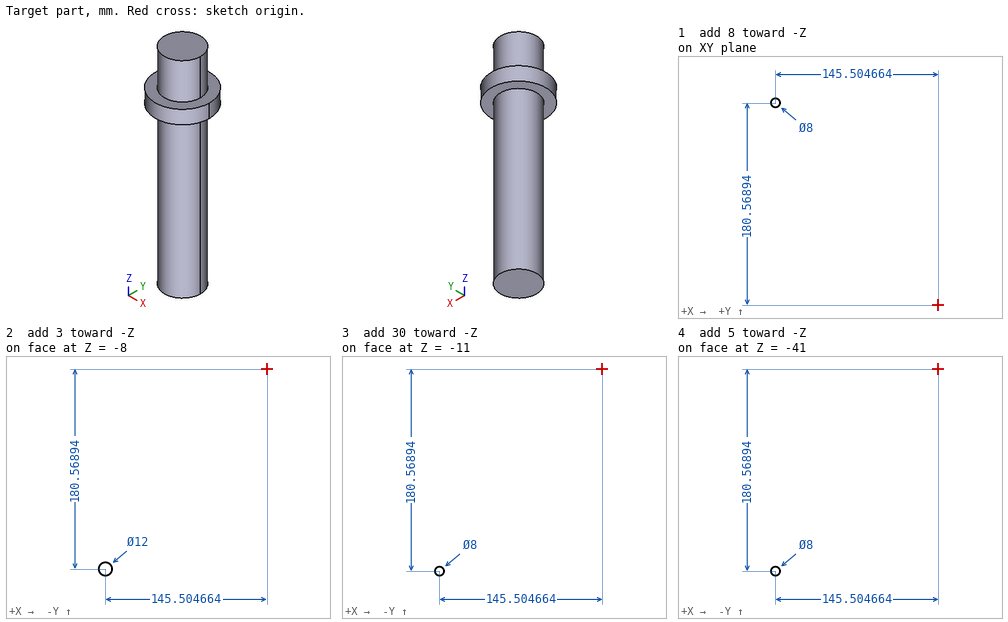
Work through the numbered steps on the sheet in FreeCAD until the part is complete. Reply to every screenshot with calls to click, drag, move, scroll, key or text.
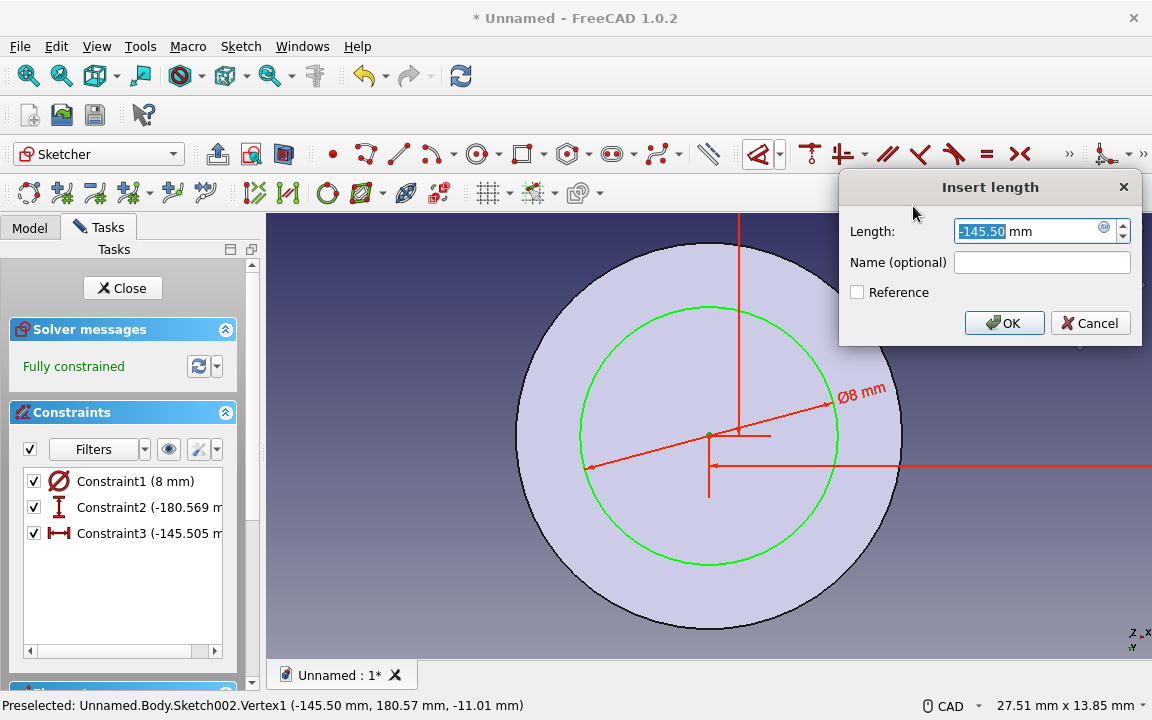
text(-145.504664)
key(Return)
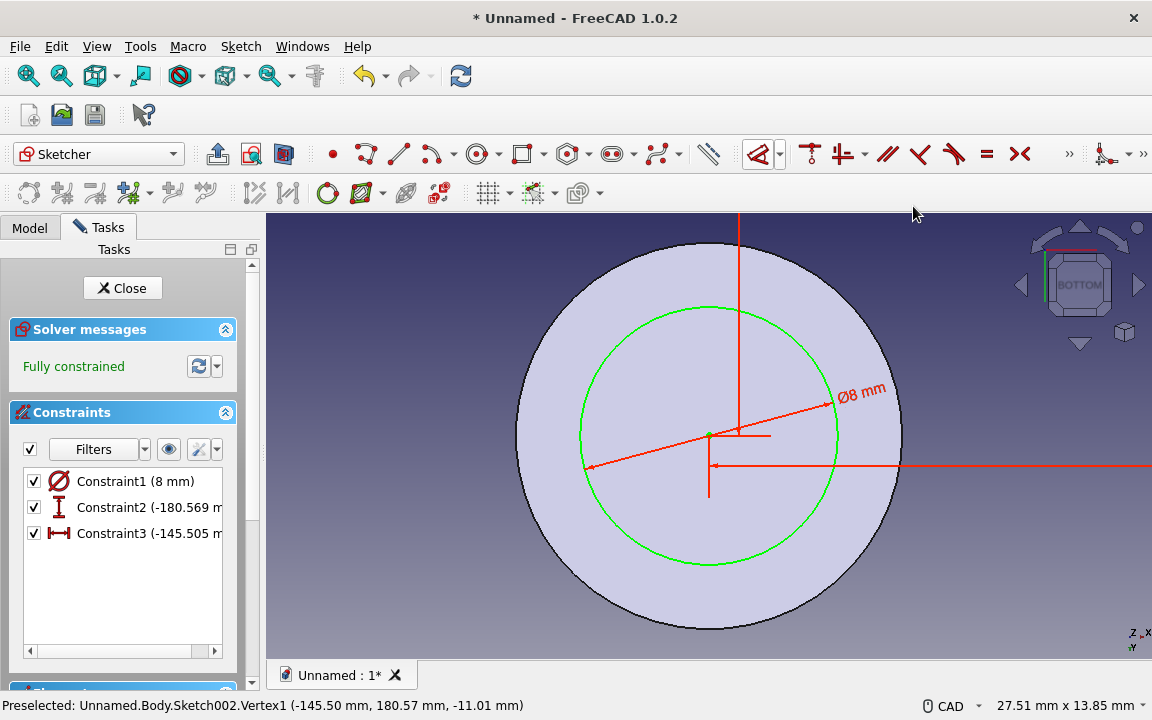
click(123, 288)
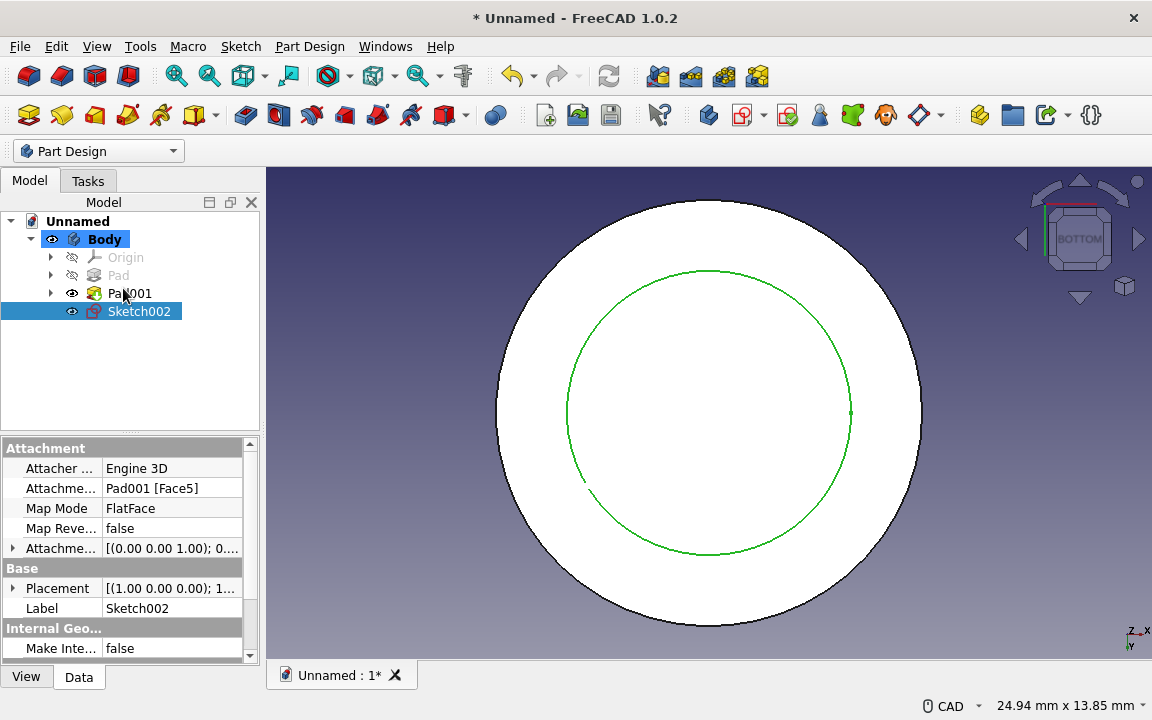
click(29, 116)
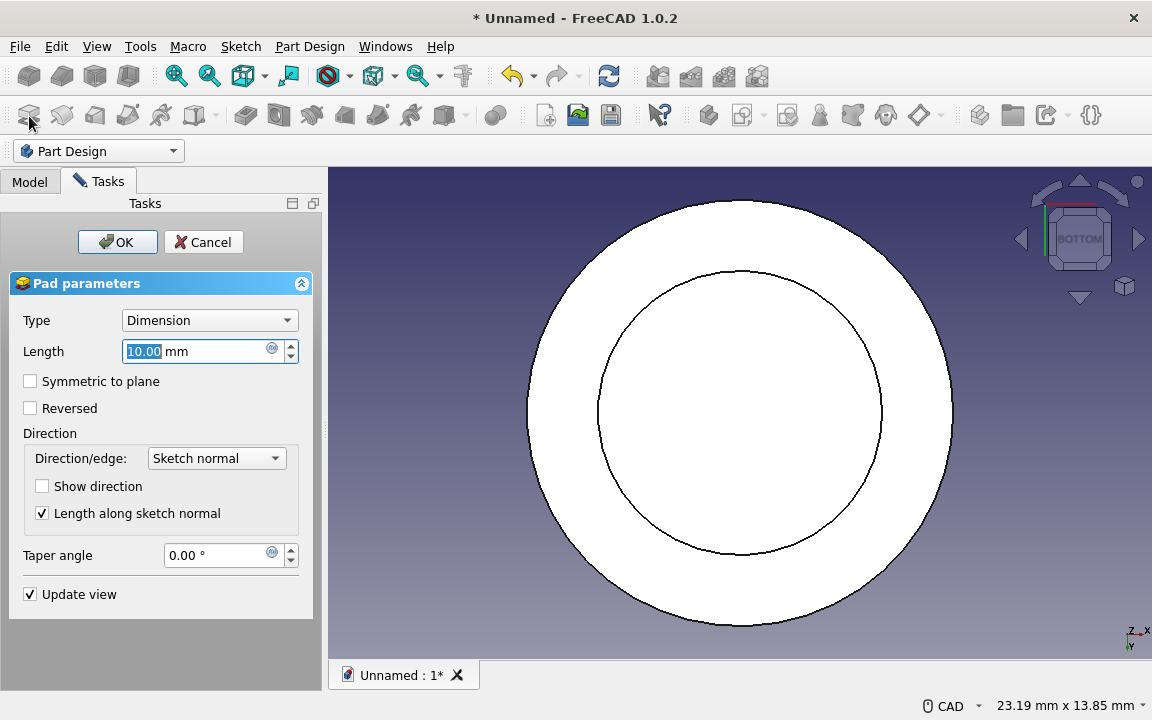
text(30)
key(Tab)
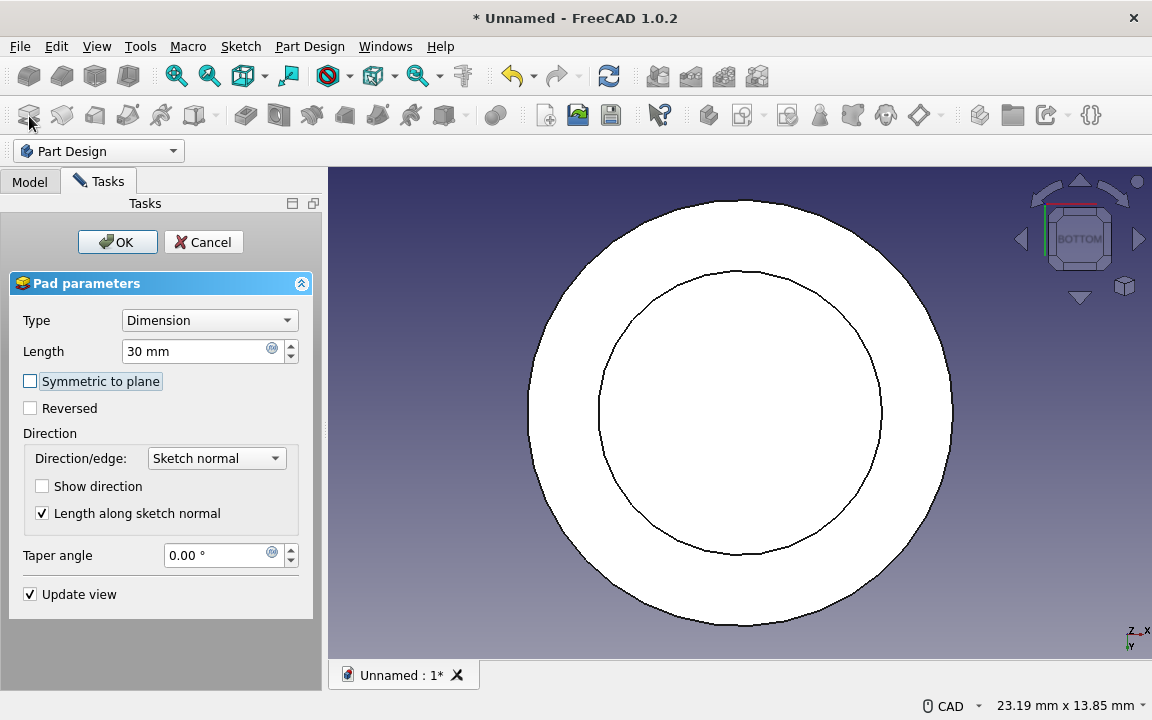
click(118, 242)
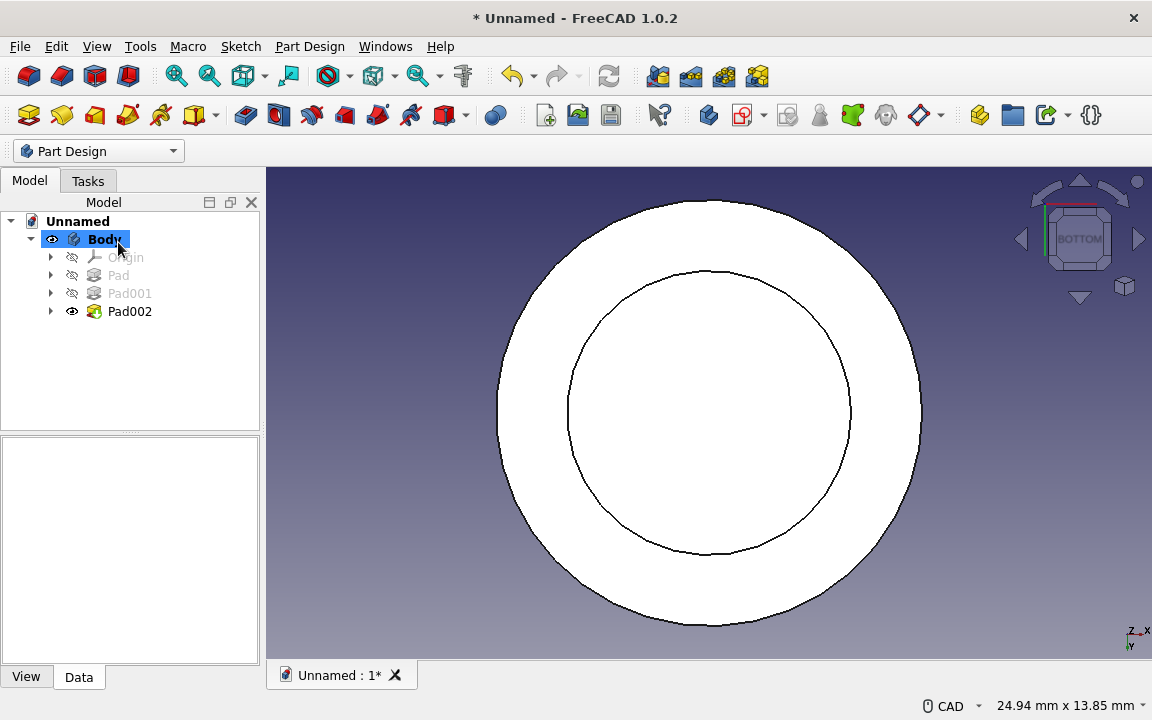
click(709, 412)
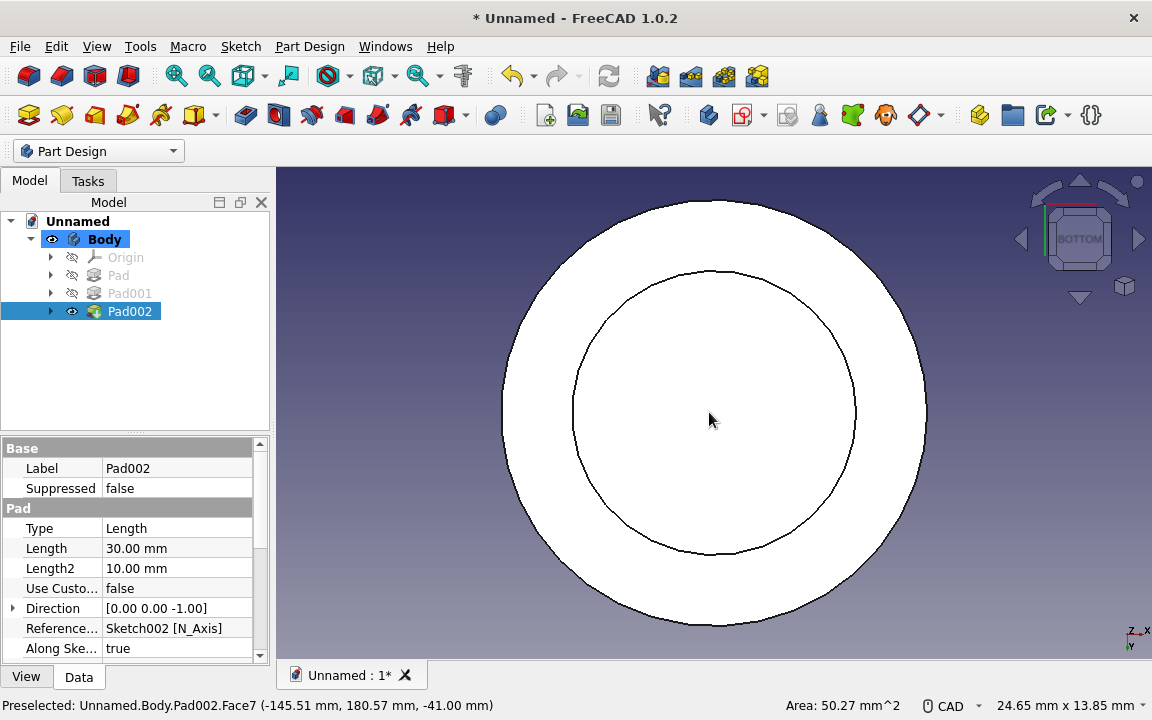
click(742, 116)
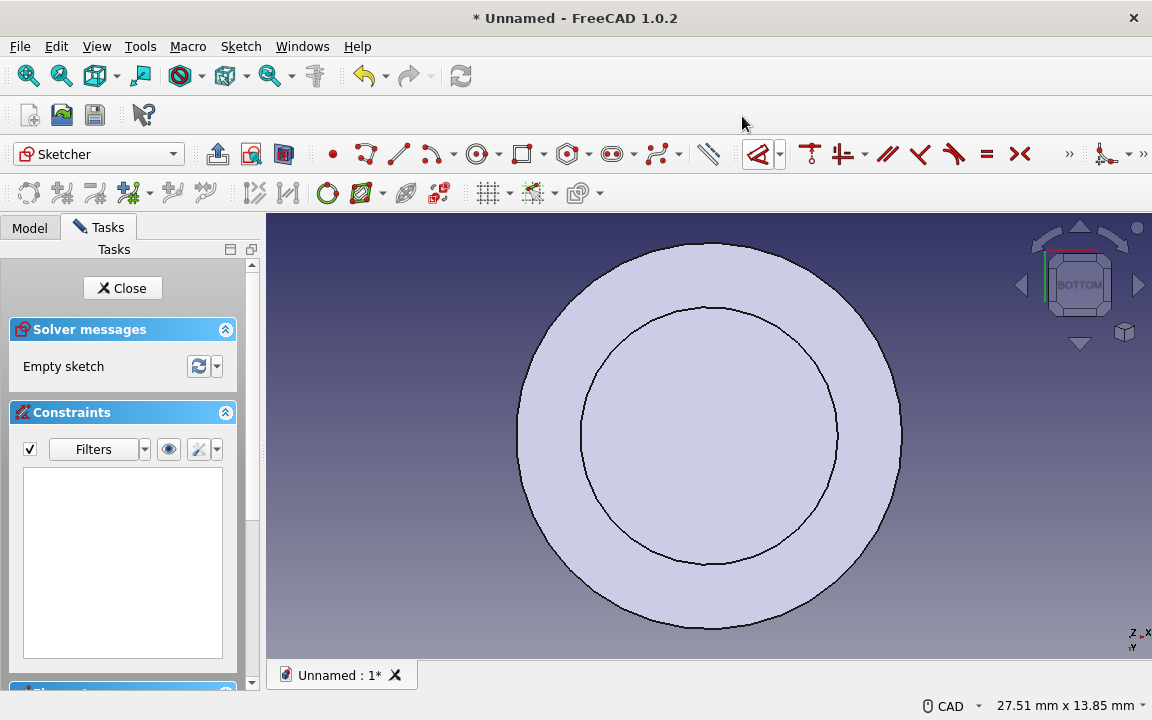
key(g)
key(c)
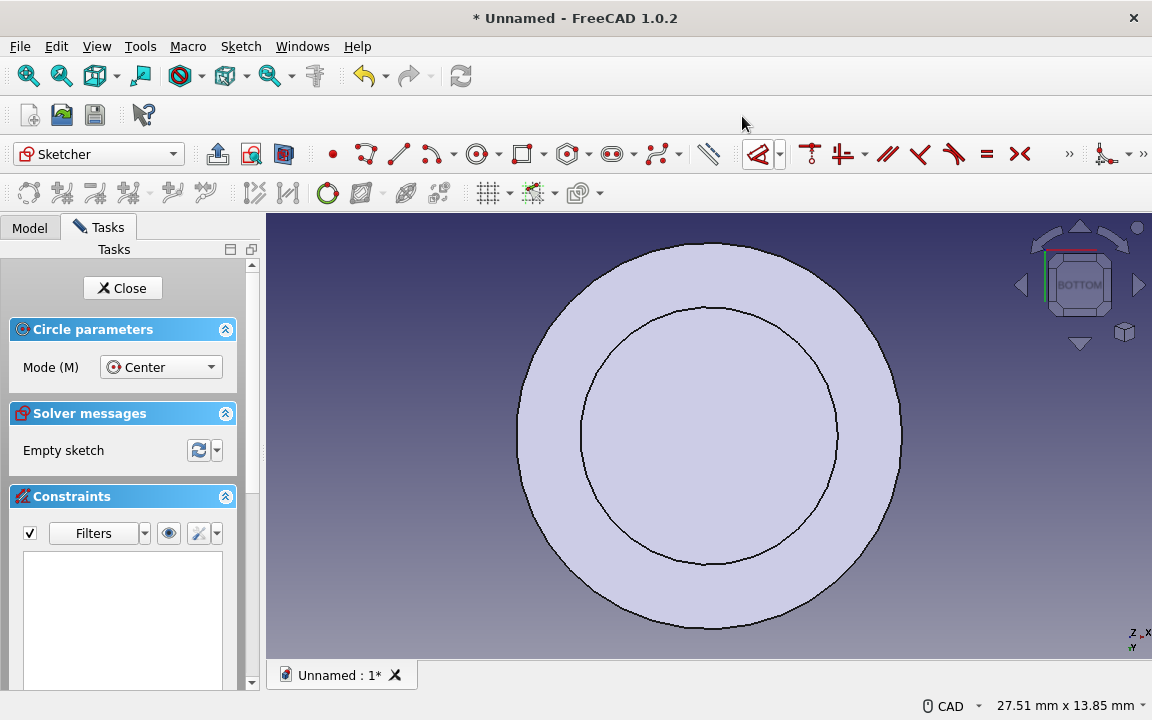
click(709, 436)
click(800, 345)
key(Escape)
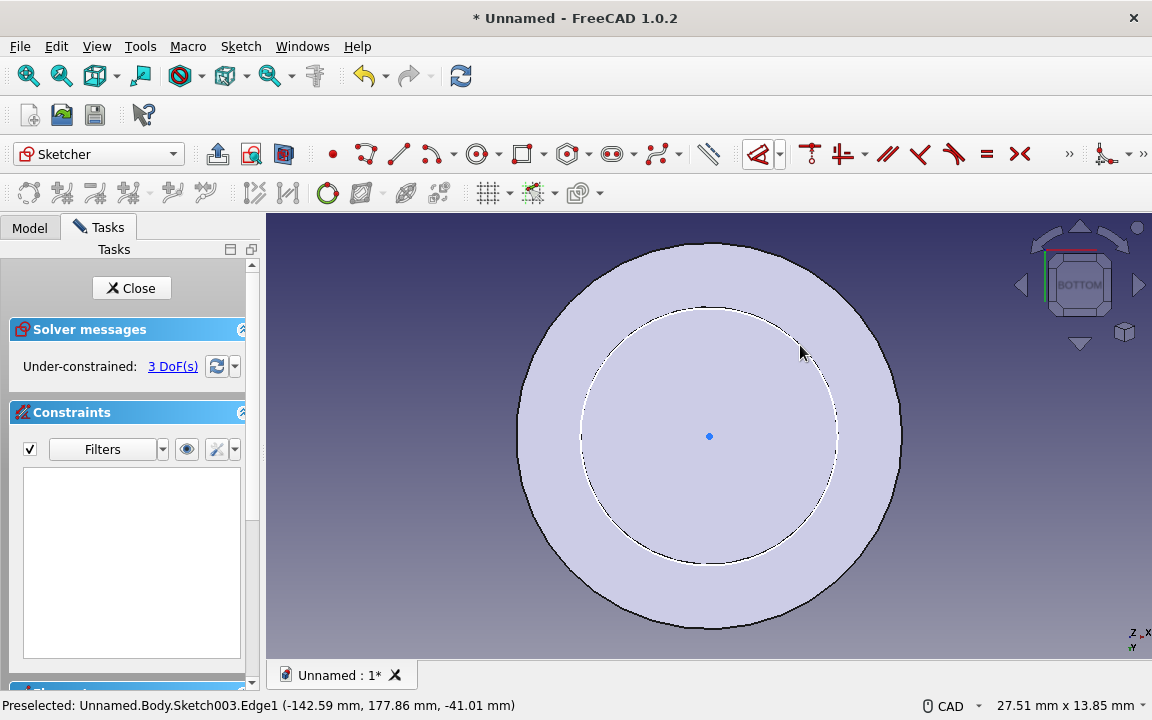
click(800, 346)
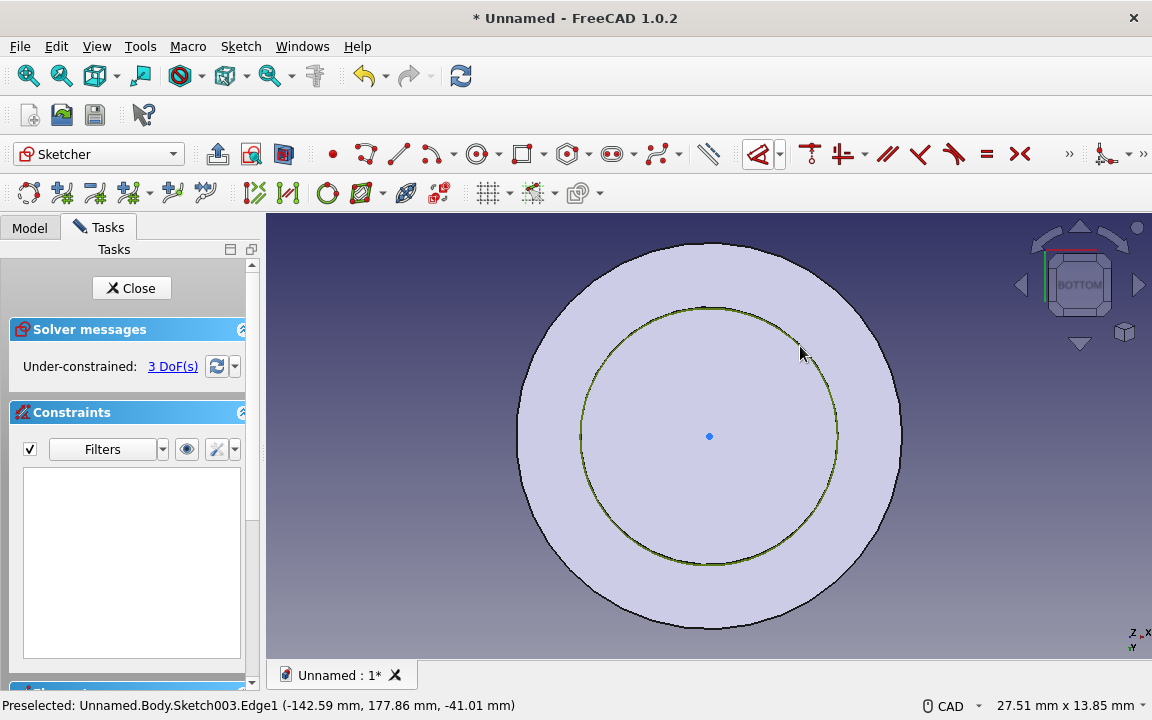
click(780, 154)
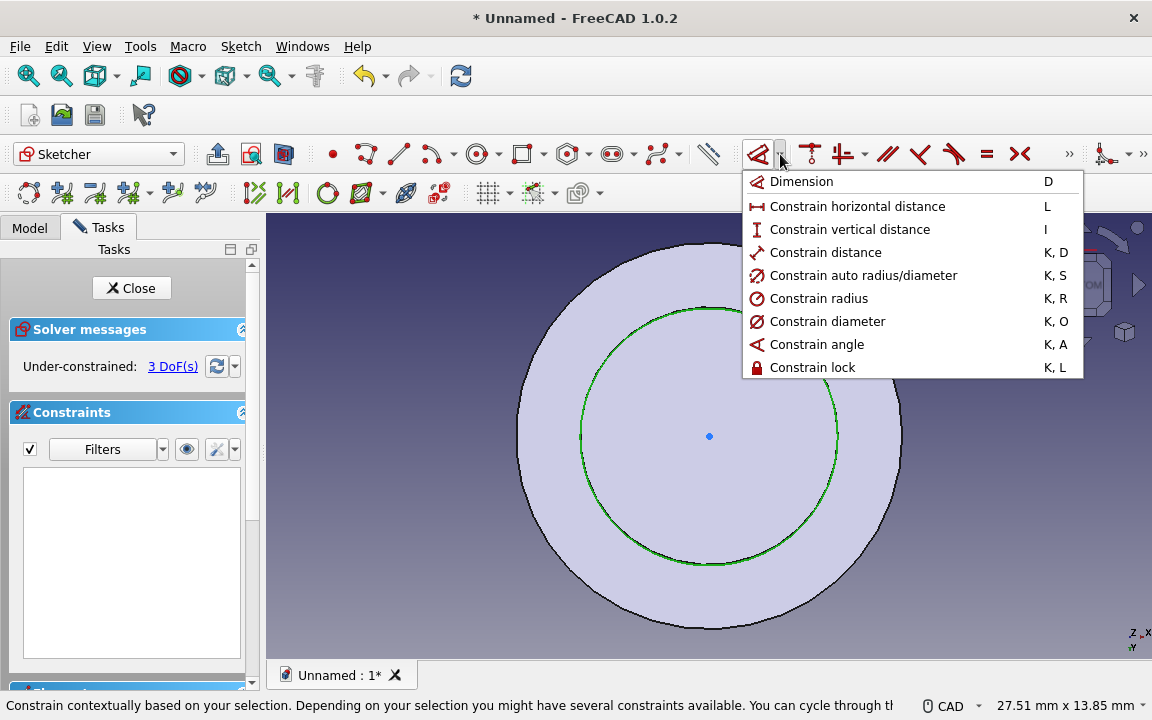
click(913, 322)